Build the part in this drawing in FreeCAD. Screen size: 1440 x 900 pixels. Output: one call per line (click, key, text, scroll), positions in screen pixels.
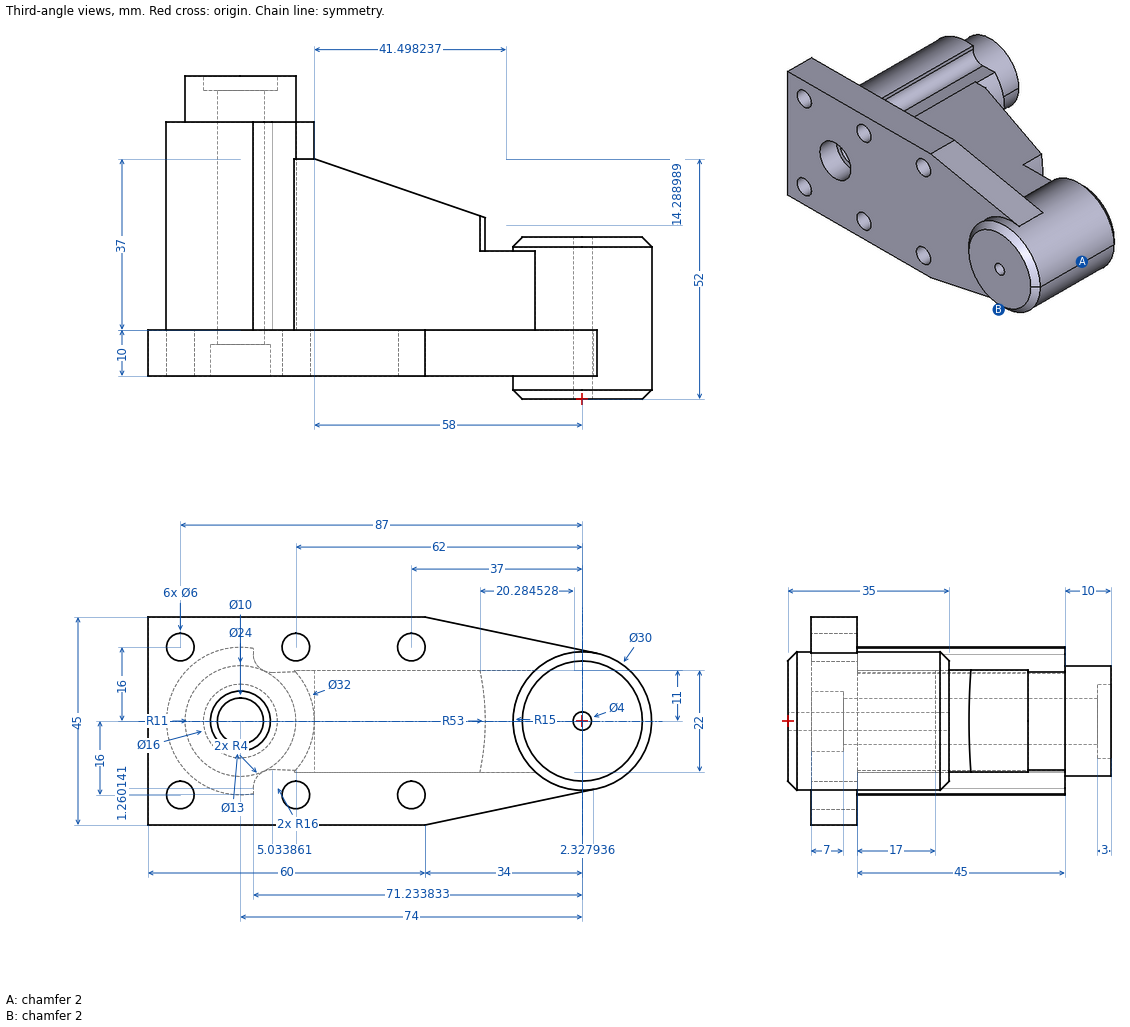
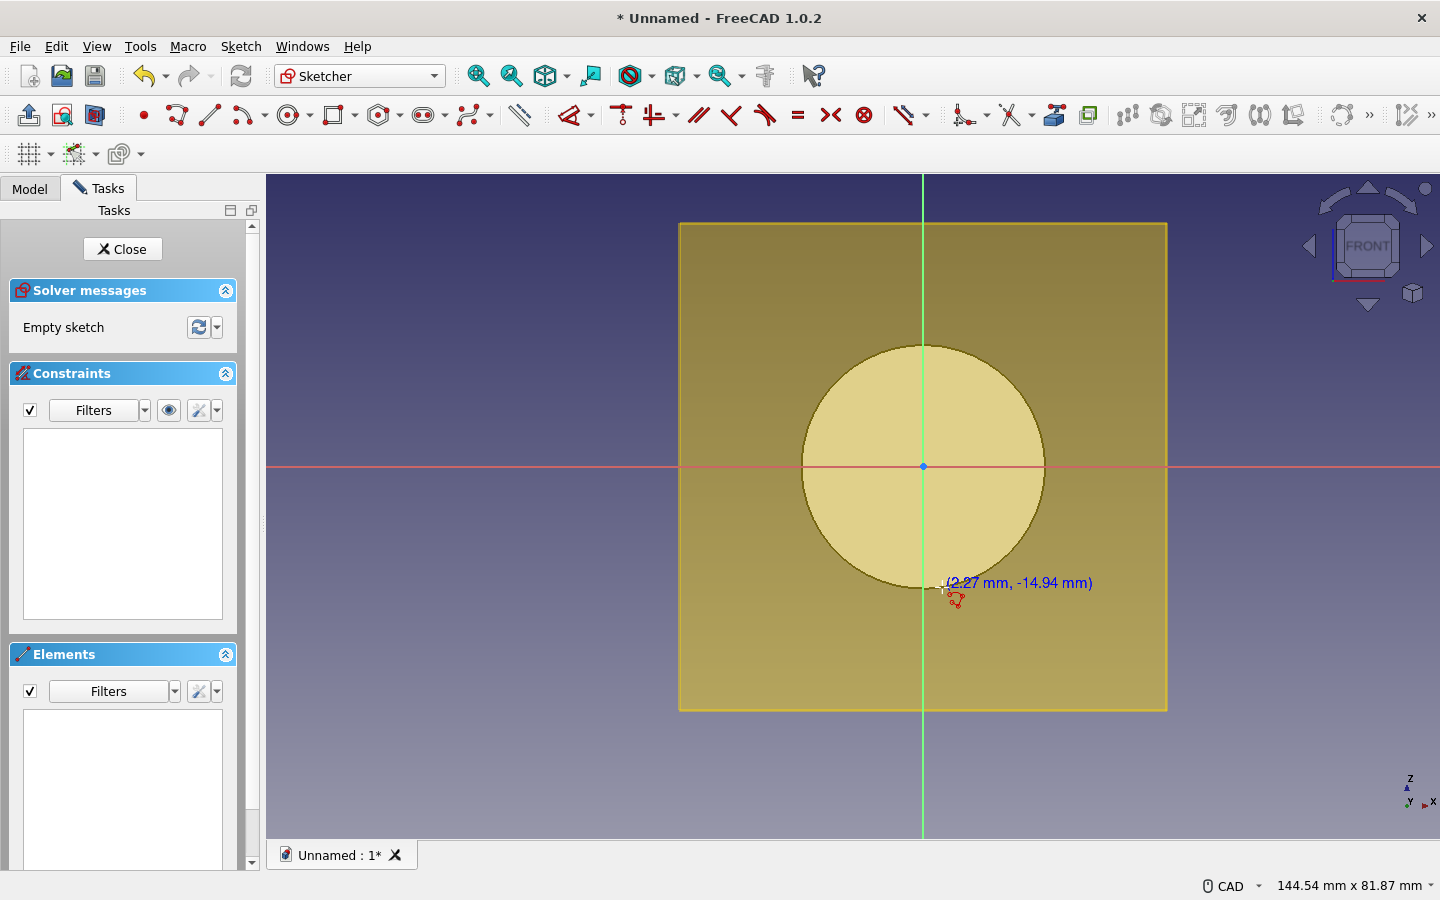
click(942, 587)
click(647, 650)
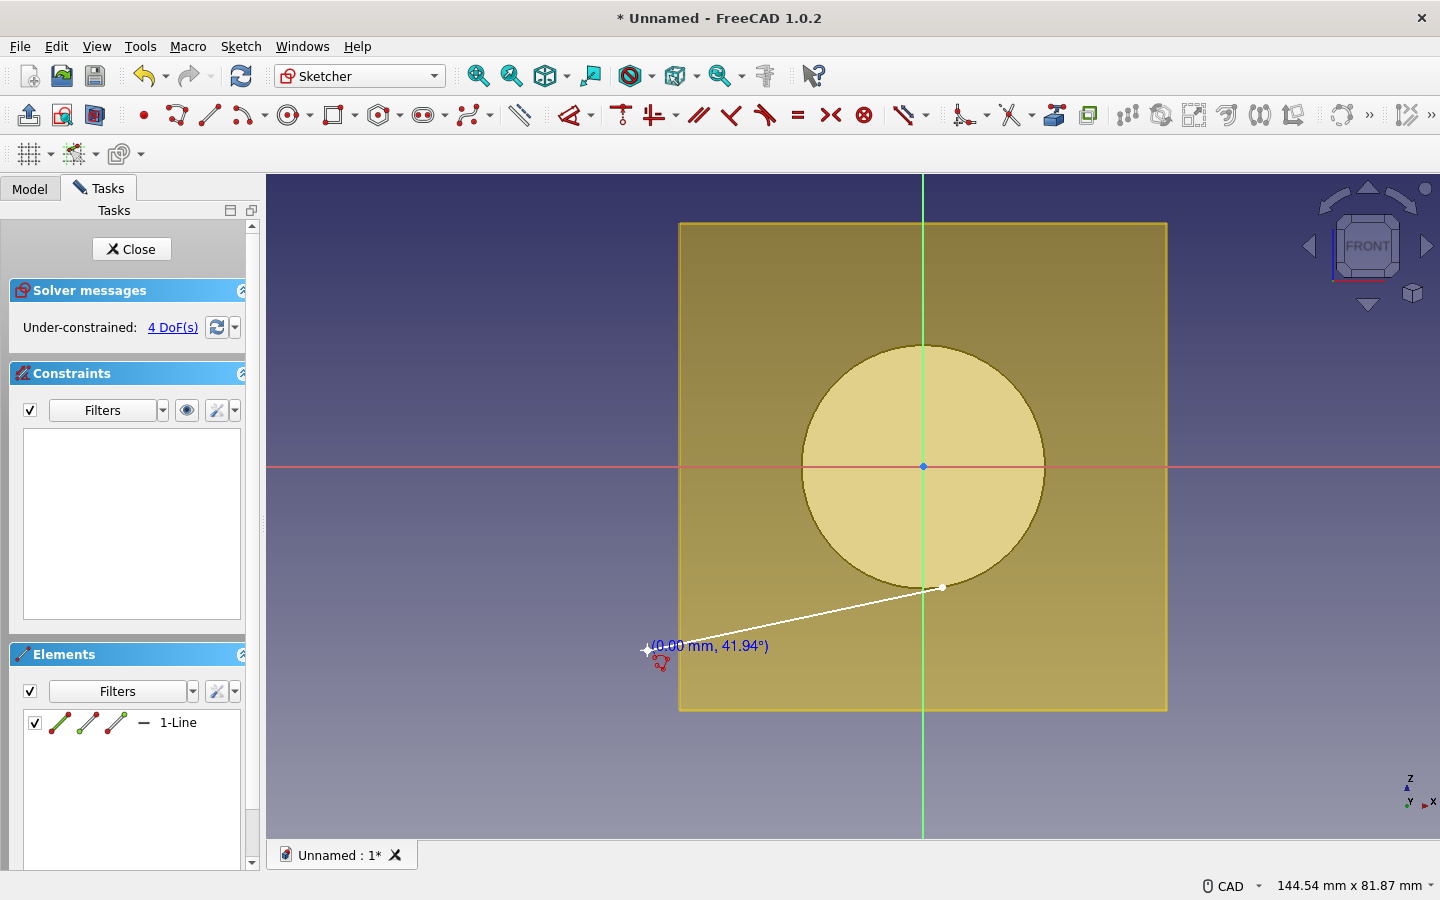
scroll(1275, 685, down, 1)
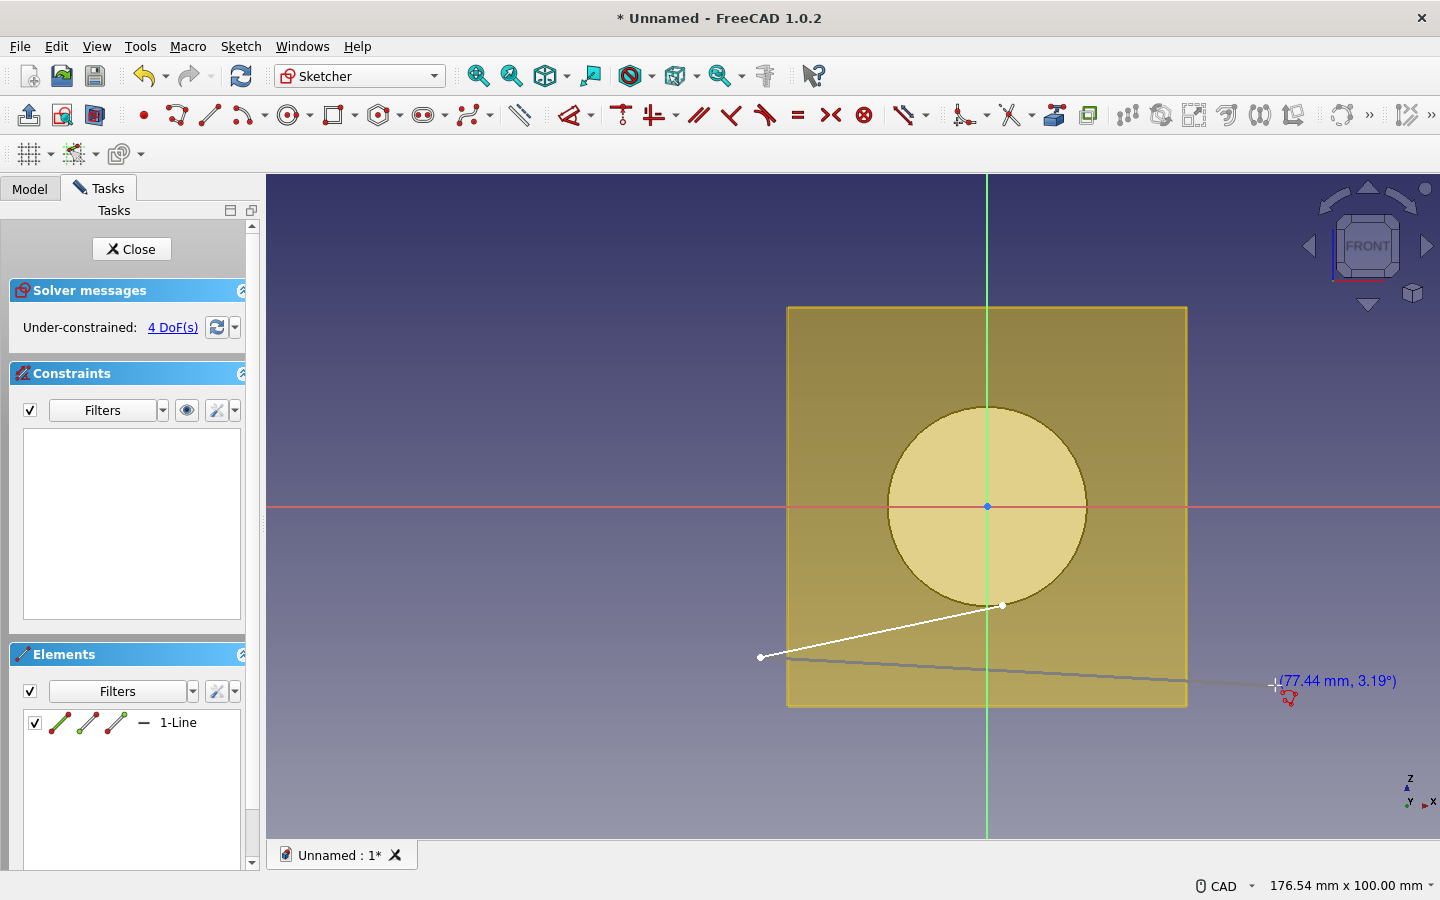
click(362, 656)
click(362, 357)
click(761, 357)
click(1008, 409)
right_click(1008, 409)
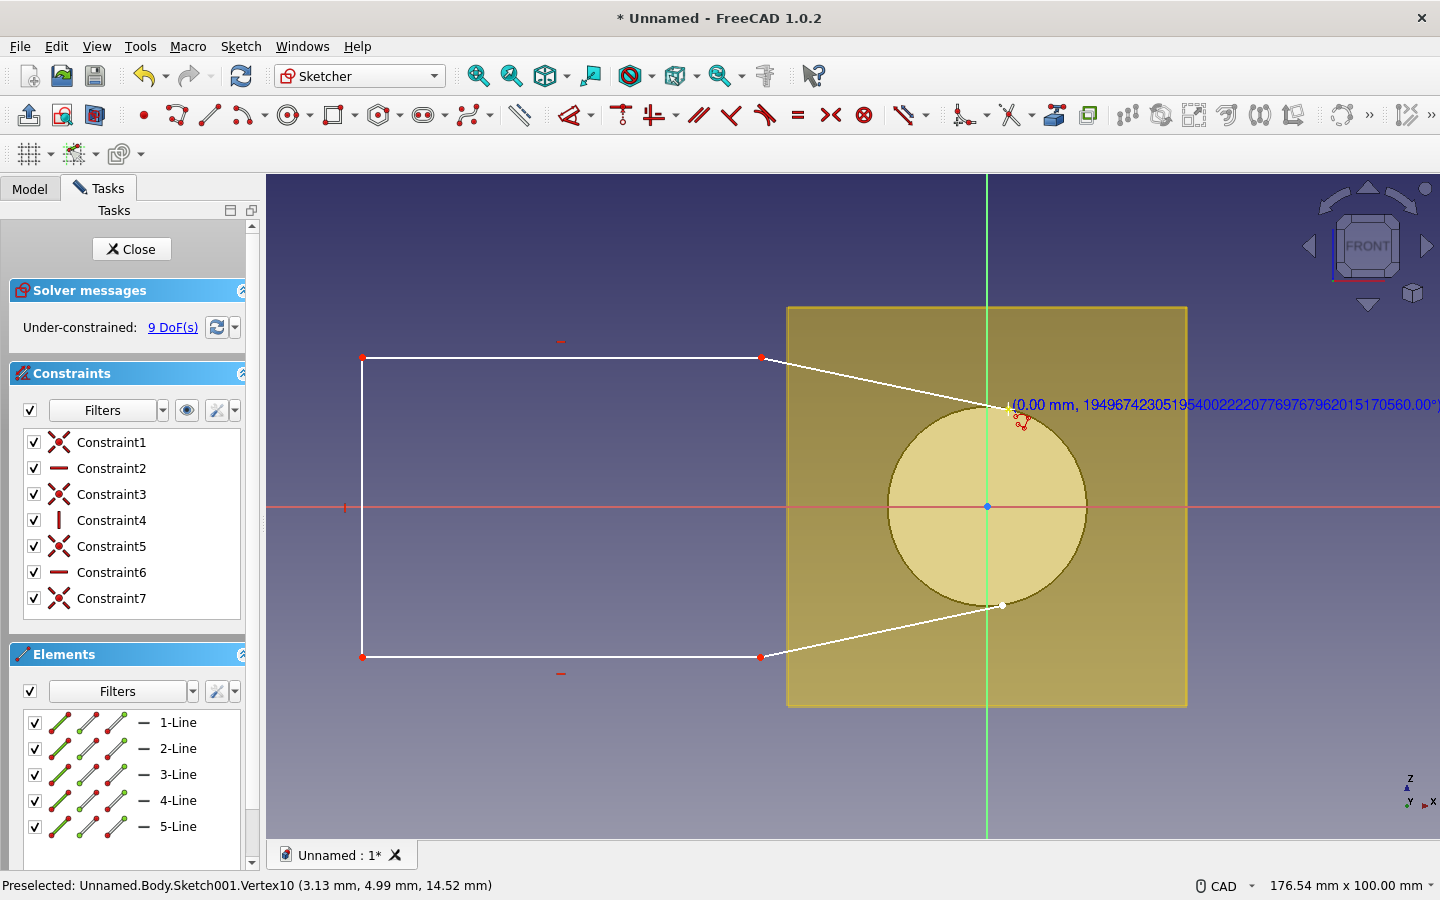
click(264, 116)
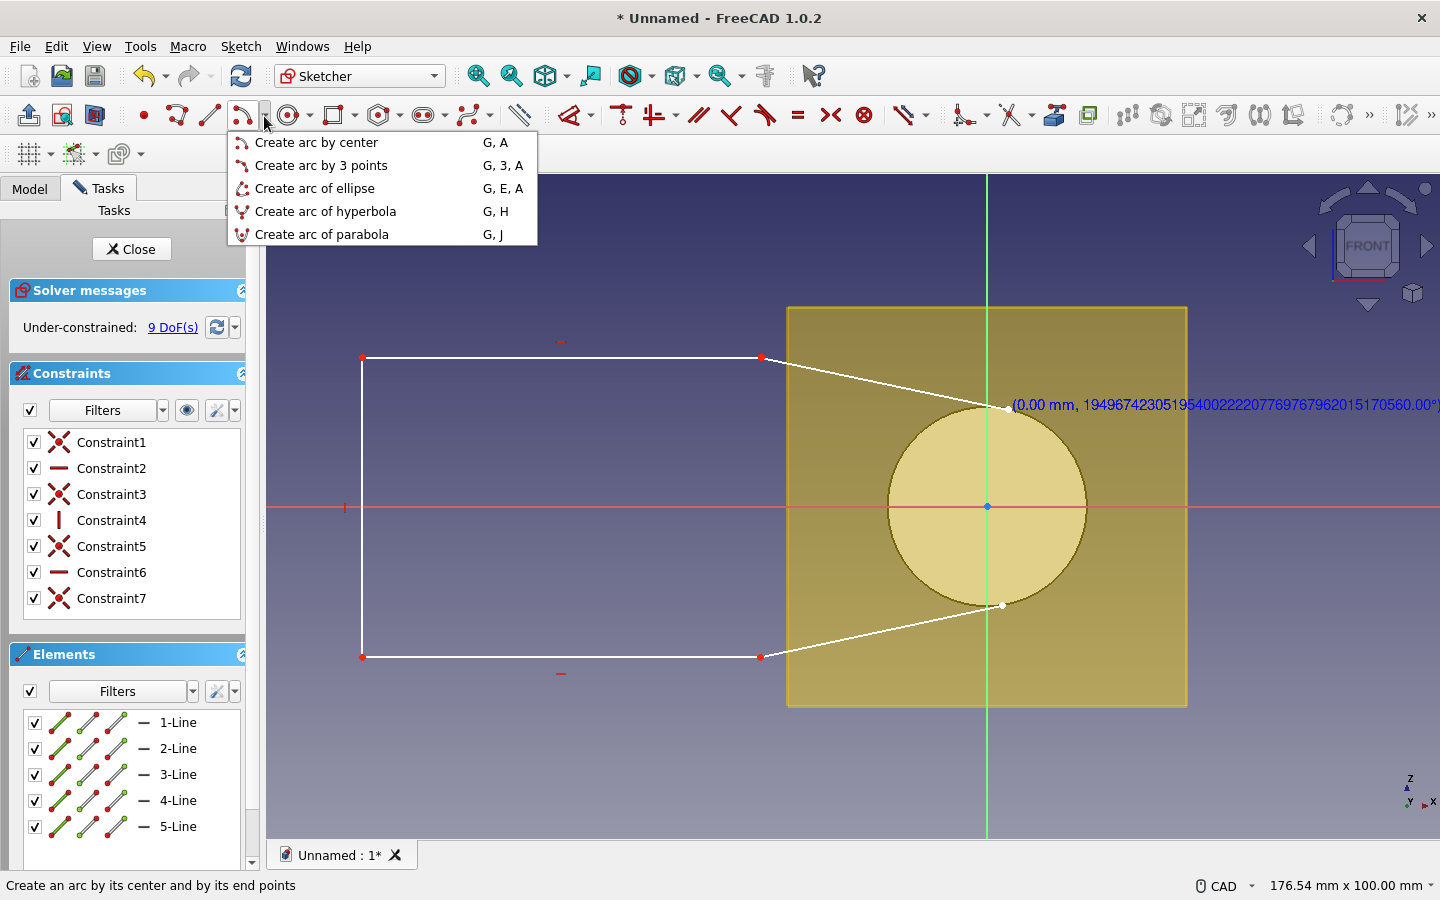
click(382, 166)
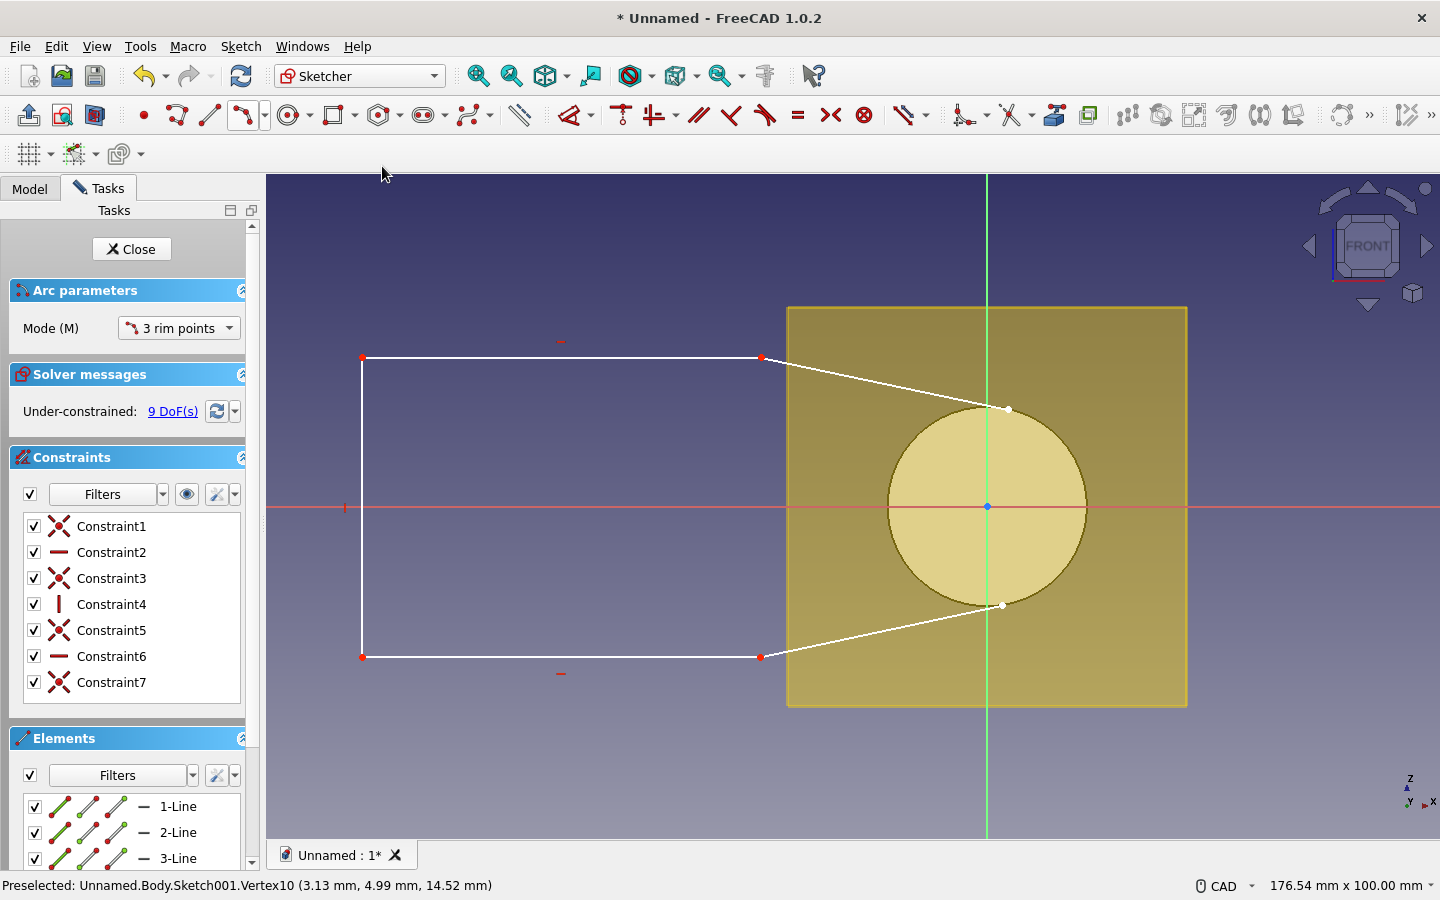
click(1008, 410)
click(1003, 606)
click(894, 470)
key(Escape)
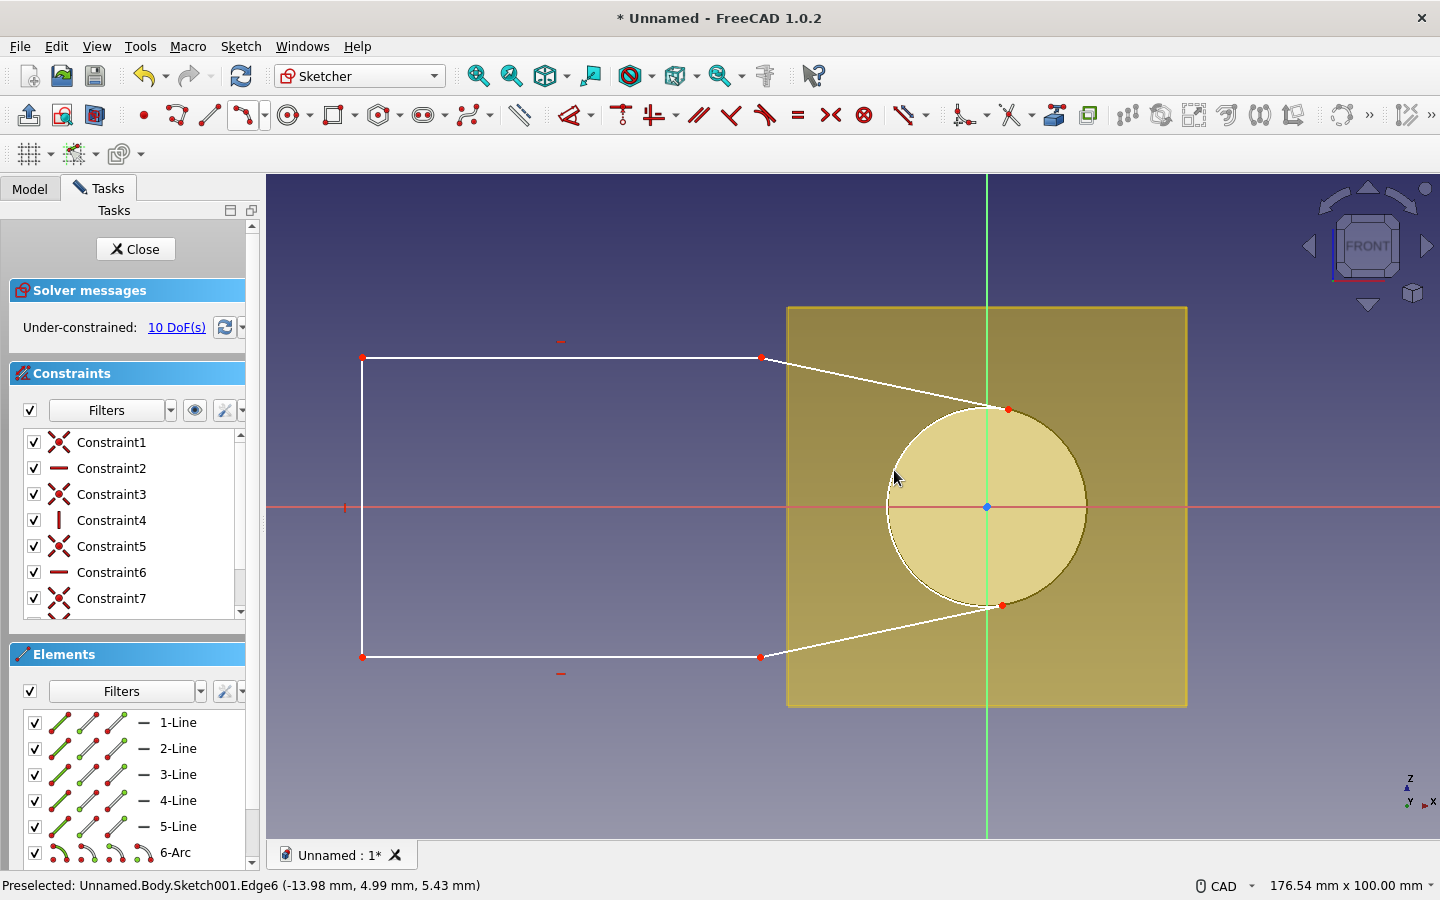
click(835, 374)